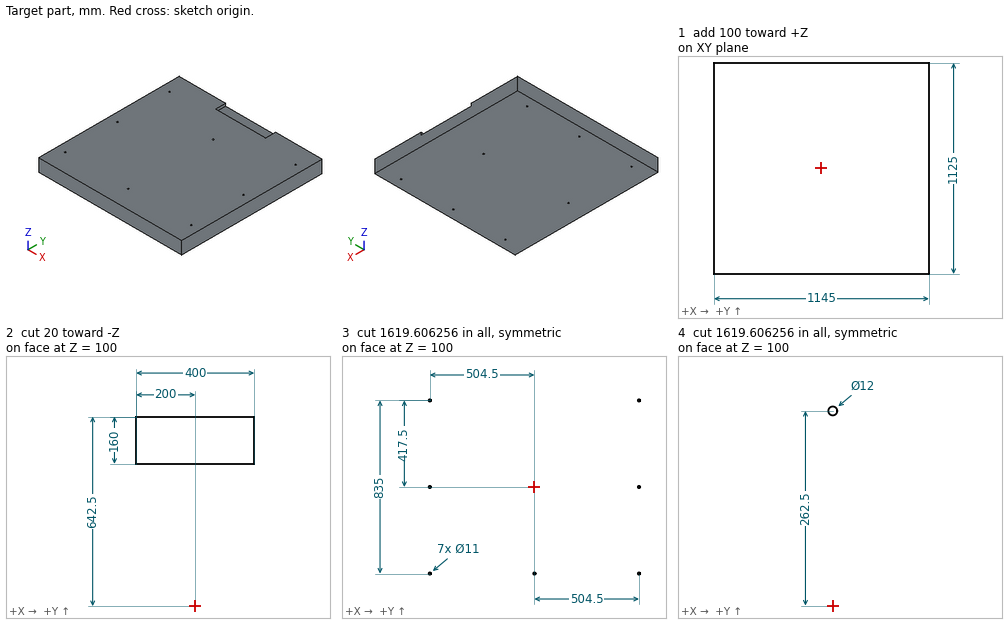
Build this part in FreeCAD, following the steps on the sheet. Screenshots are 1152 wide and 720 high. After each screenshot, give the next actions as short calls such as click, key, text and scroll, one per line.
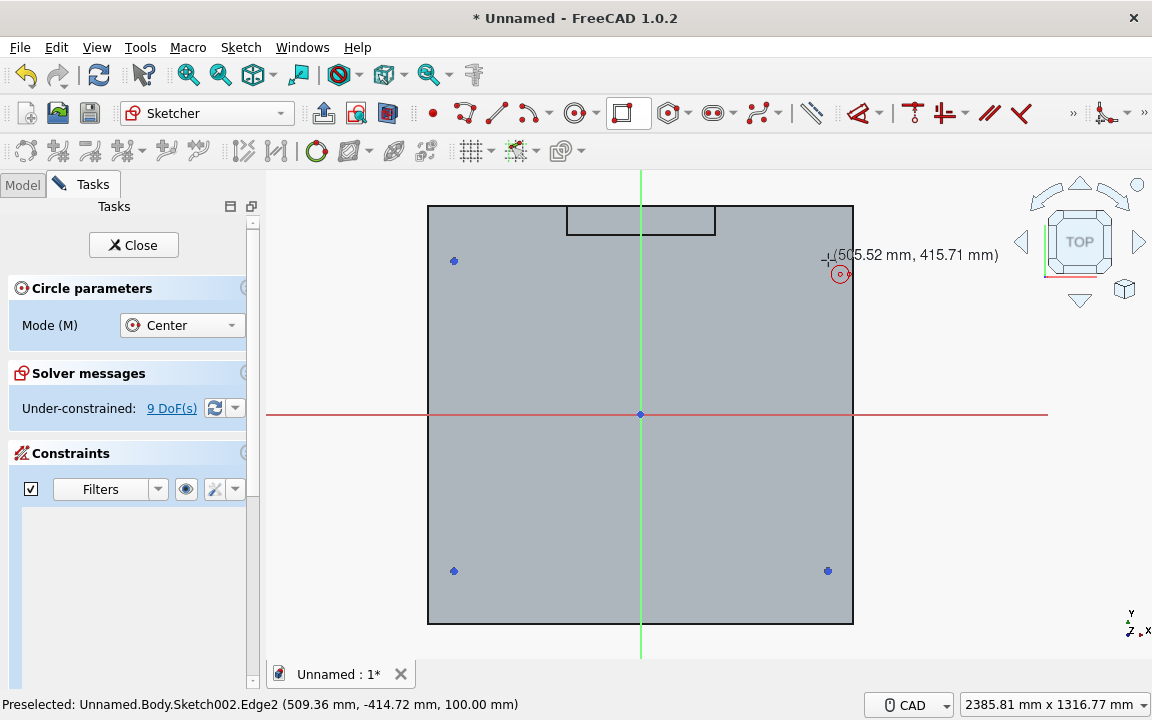
click(828, 260)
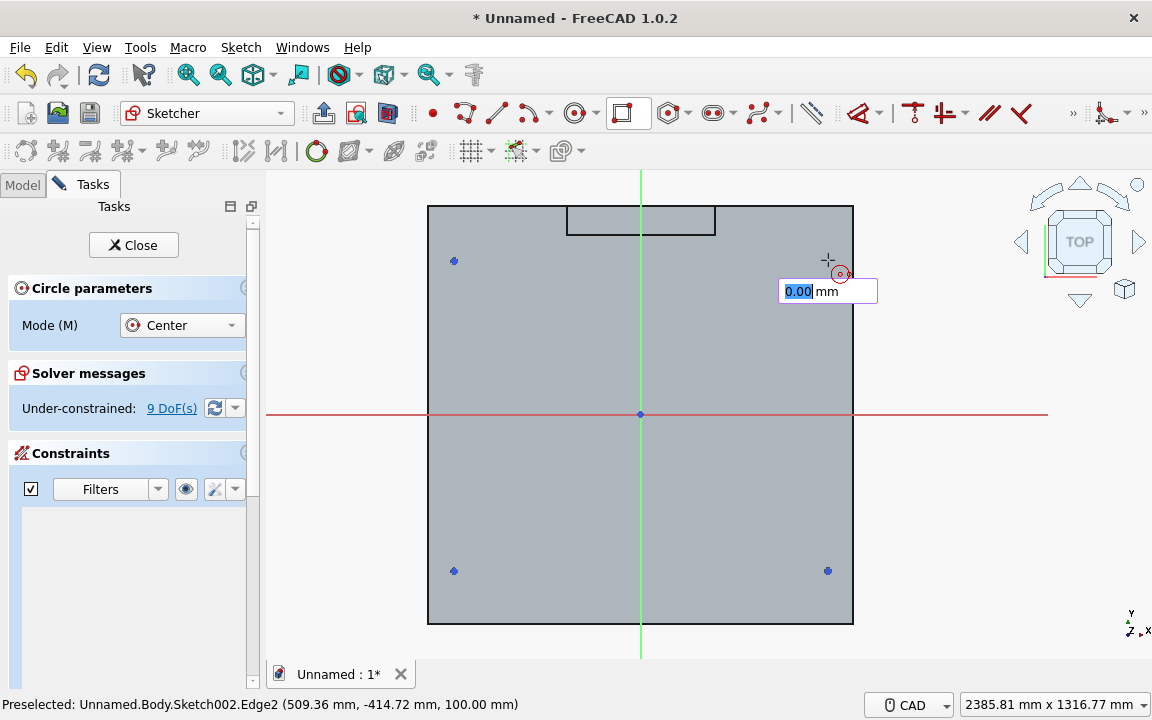
scroll(830, 258, up, 11)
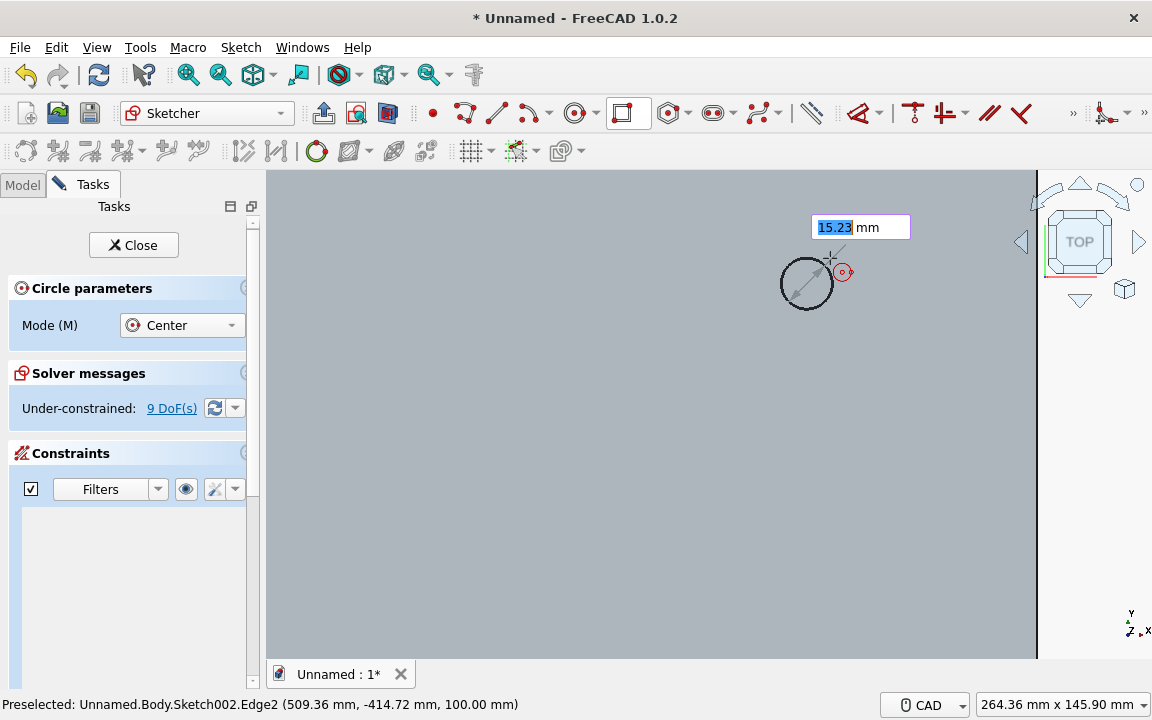
click(822, 258)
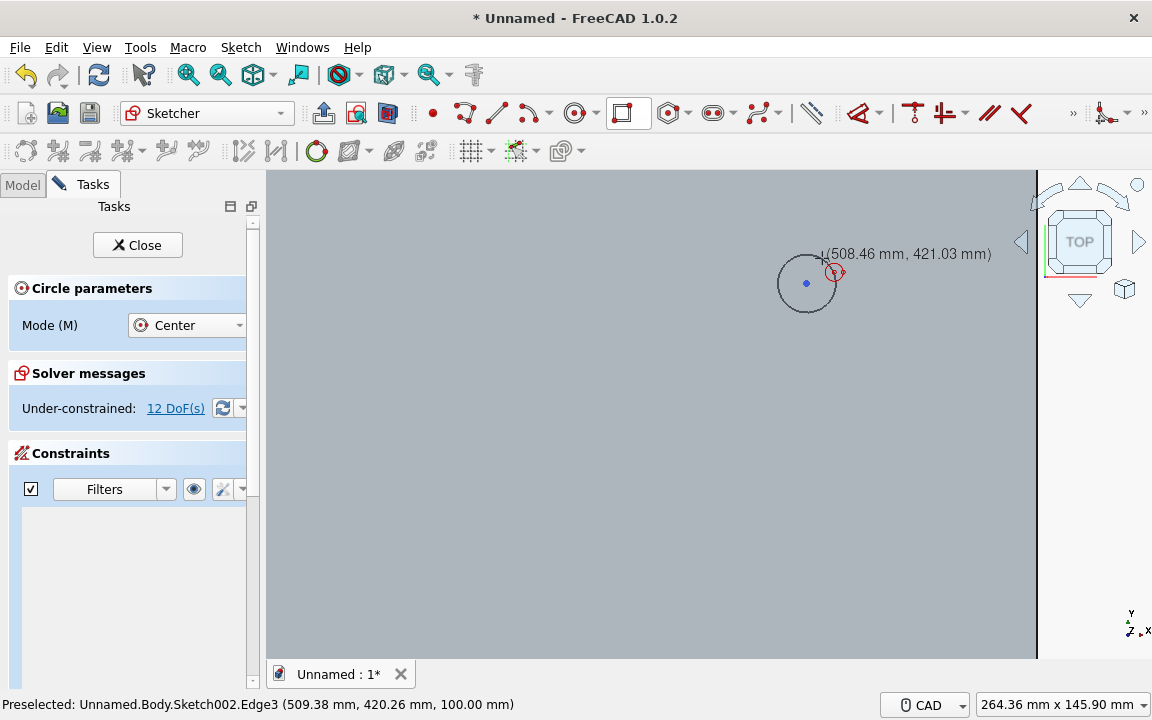
scroll(830, 258, down, 11)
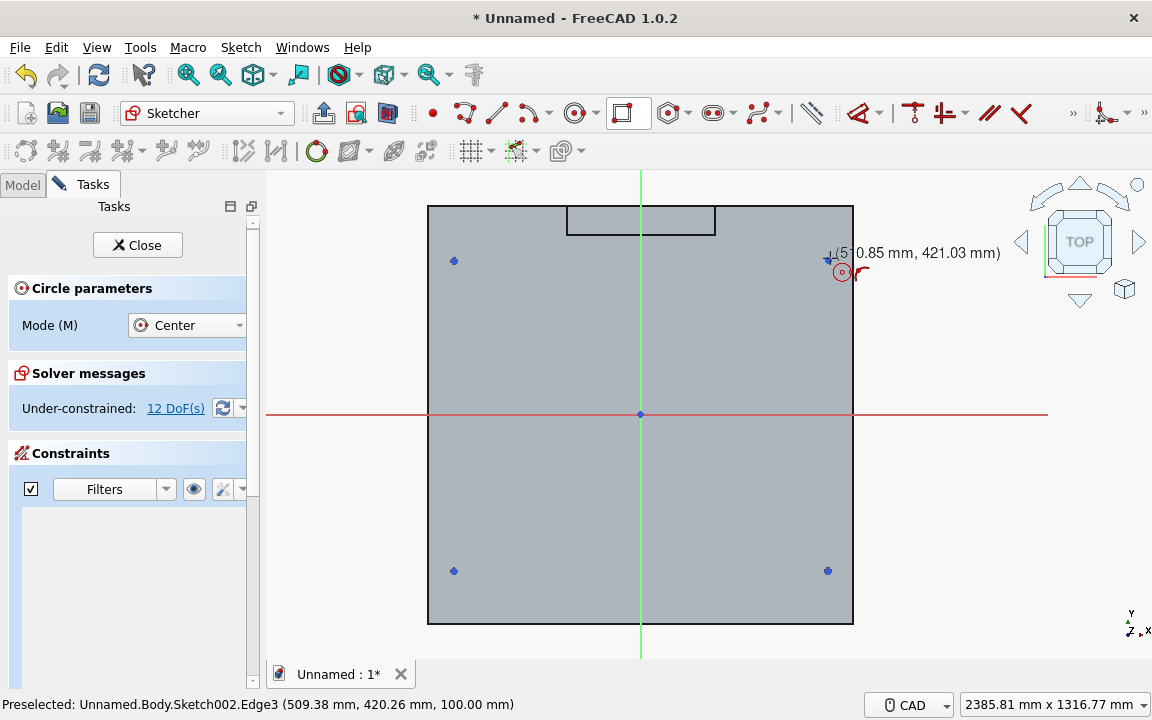
scroll(641, 570, up, 13)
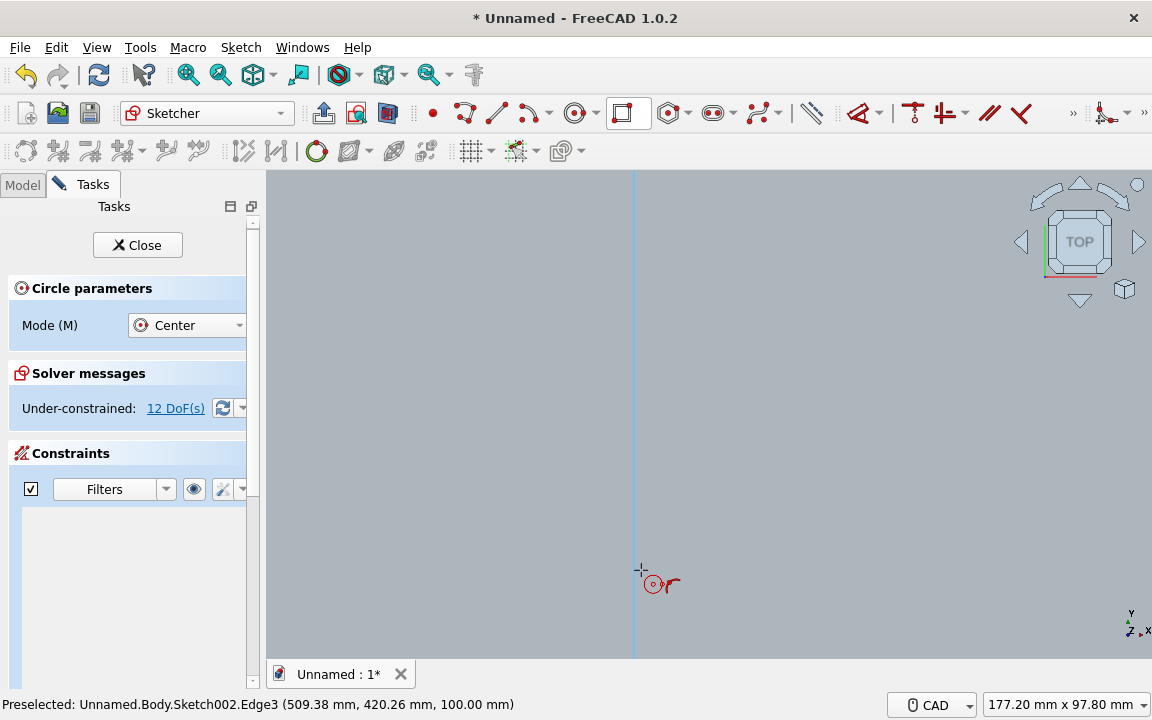
scroll(641, 571, down, 13)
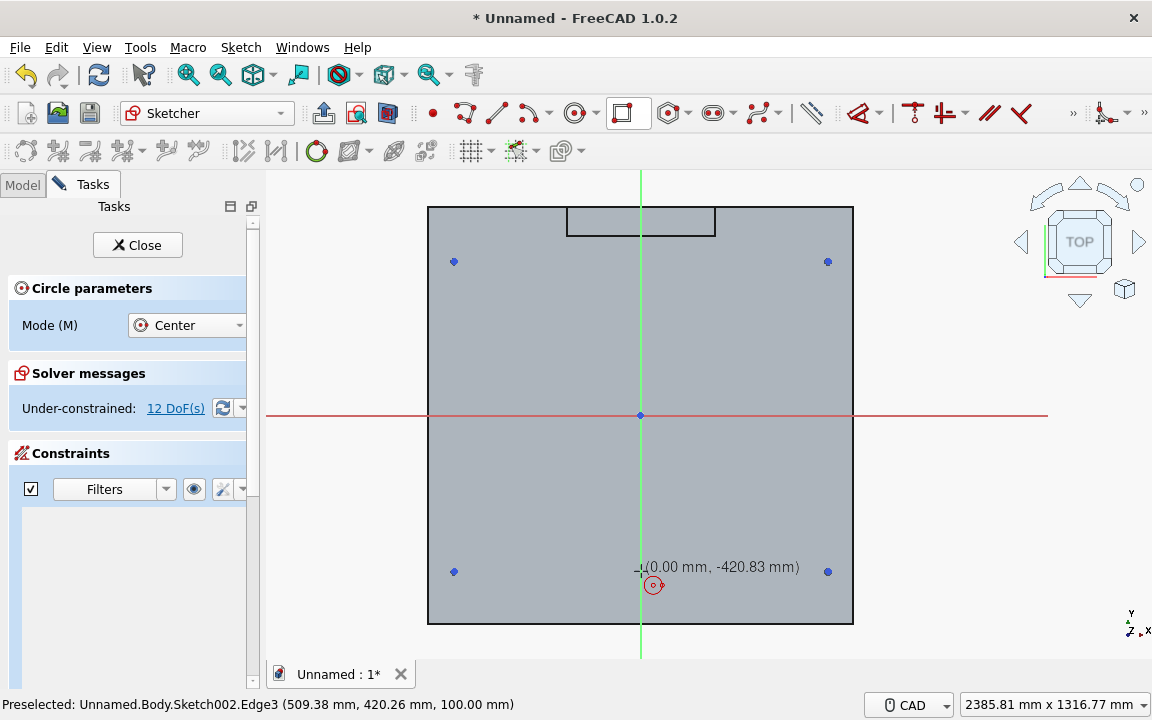
click(641, 571)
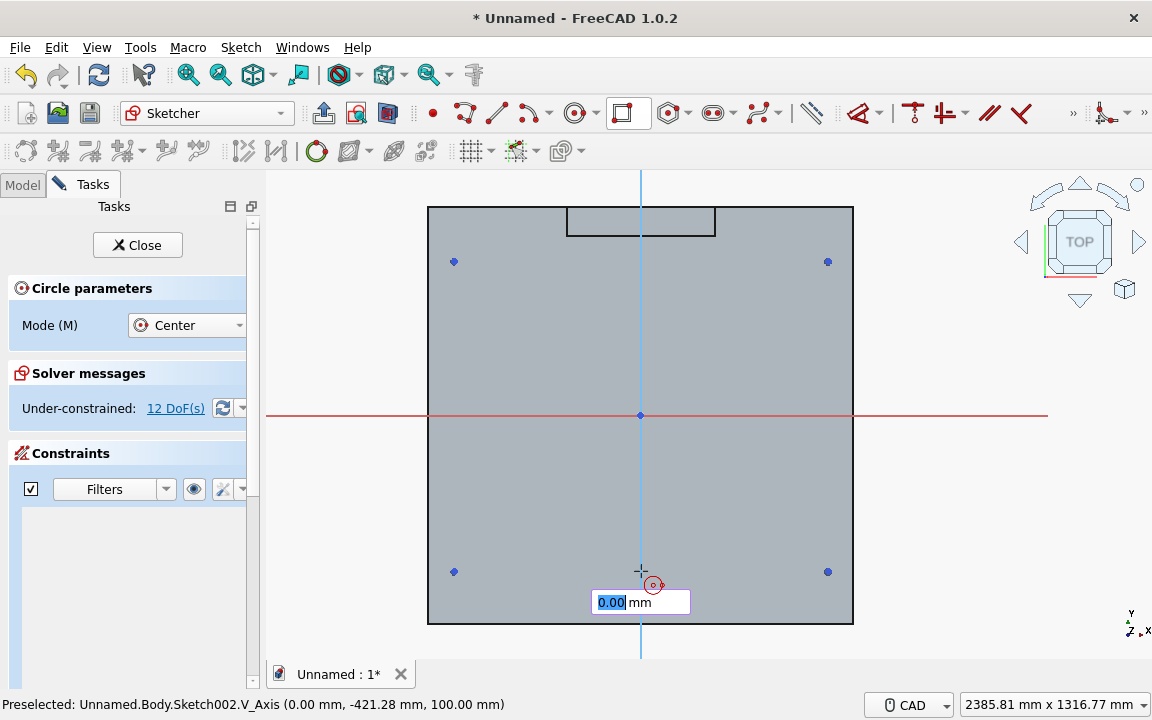
scroll(643, 570, up, 11)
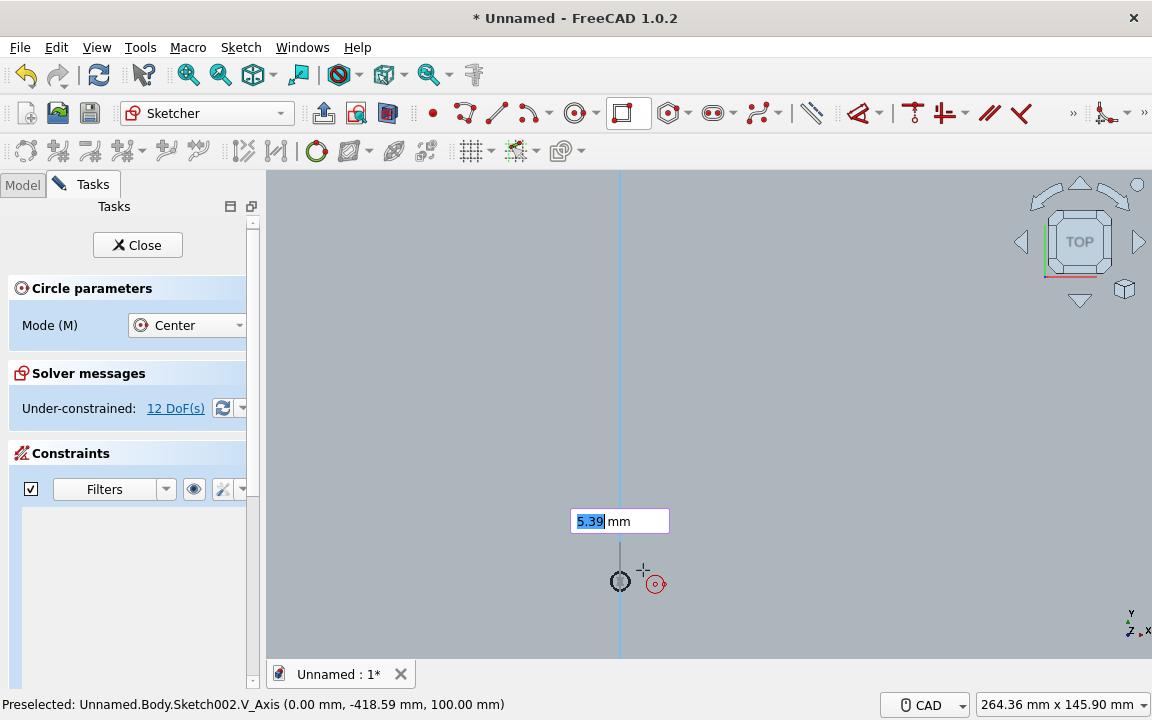
click(638, 563)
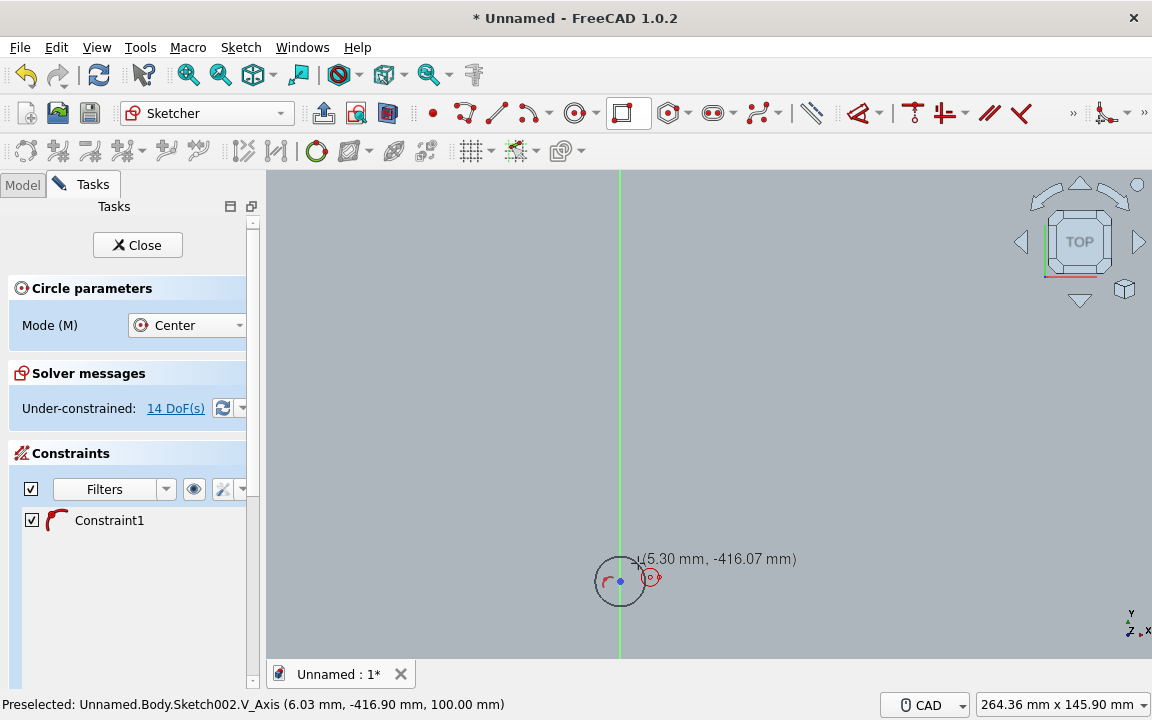
scroll(643, 570, down, 11)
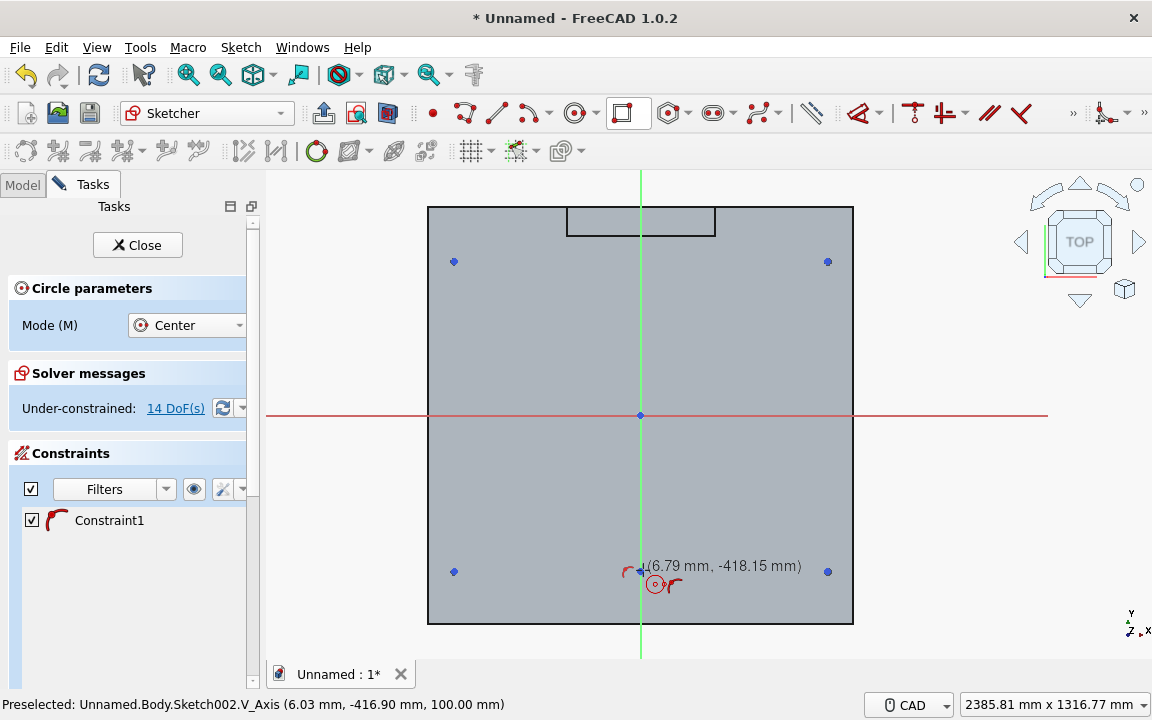
scroll(454, 416, up, 13)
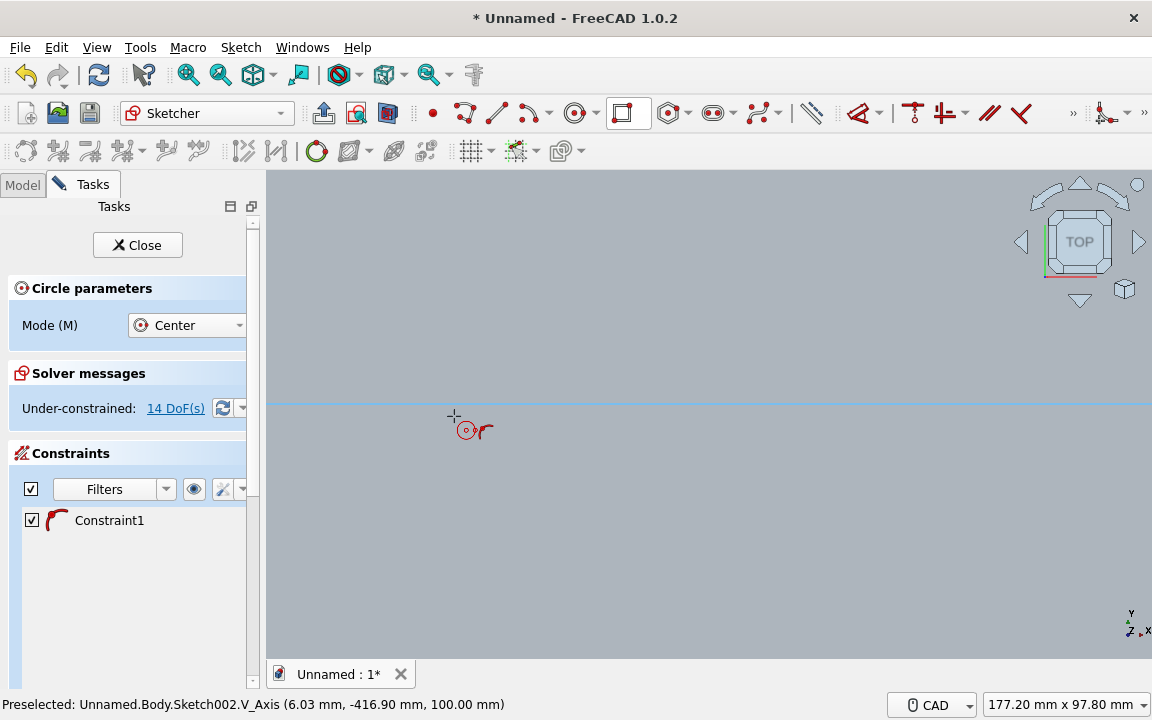
scroll(454, 415, down, 13)